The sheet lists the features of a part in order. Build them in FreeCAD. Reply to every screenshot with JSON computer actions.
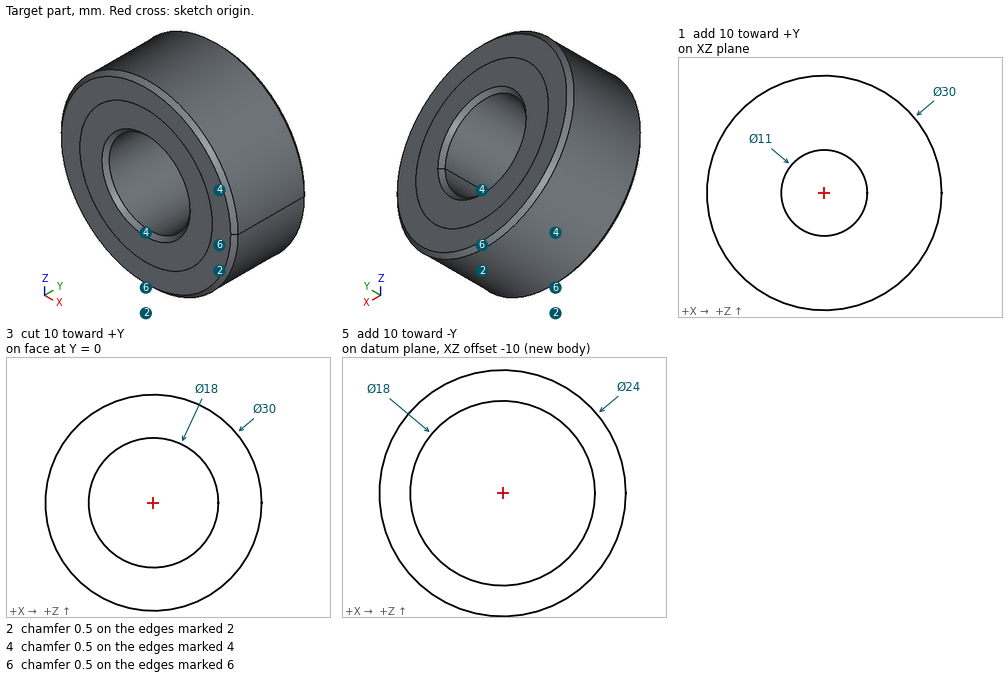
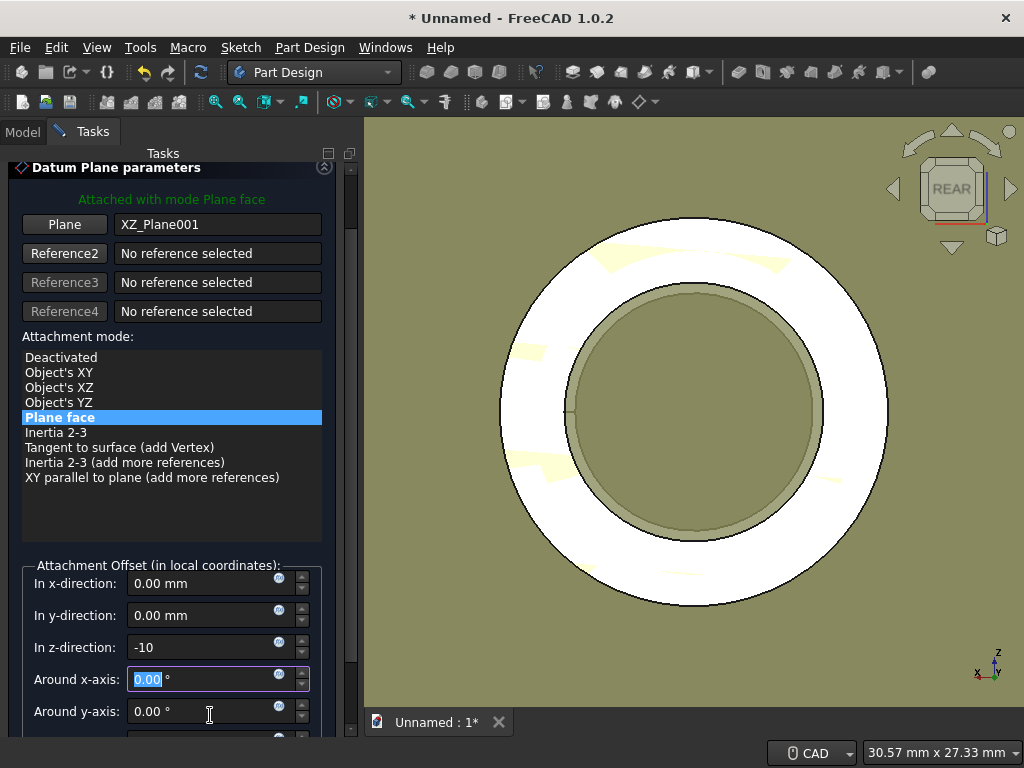
{"action": "scroll", "coordinate": [351, 450], "scroll_direction": "up", "scroll_amount": 2}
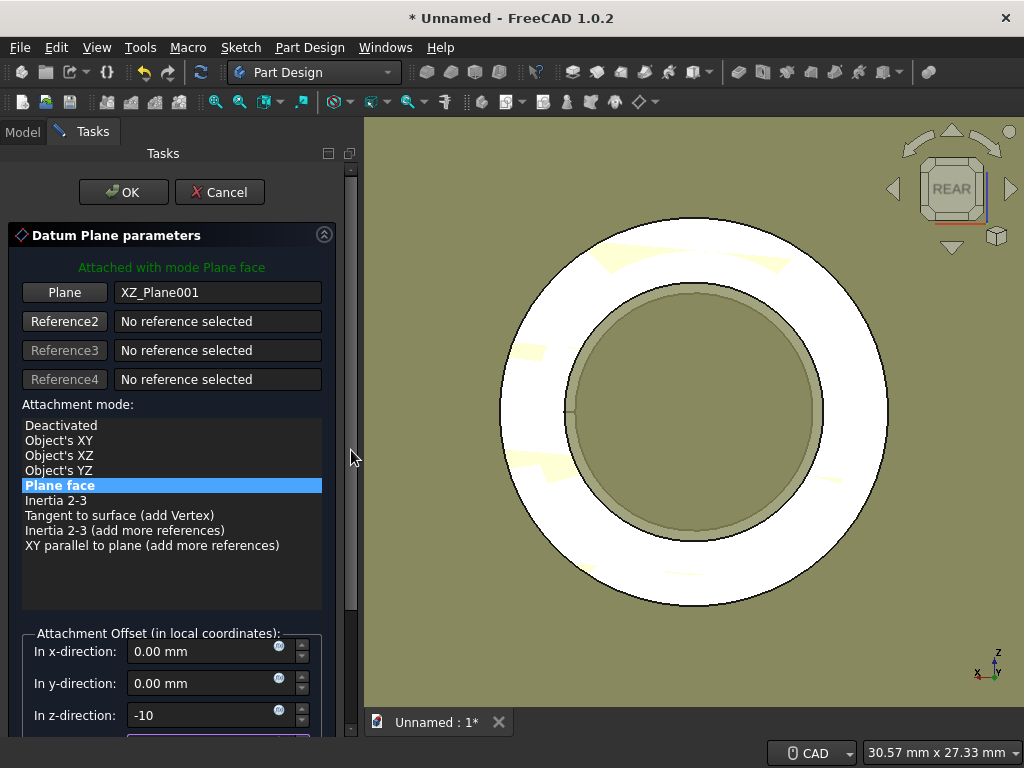
{"action": "left_click", "coordinate": [124, 192]}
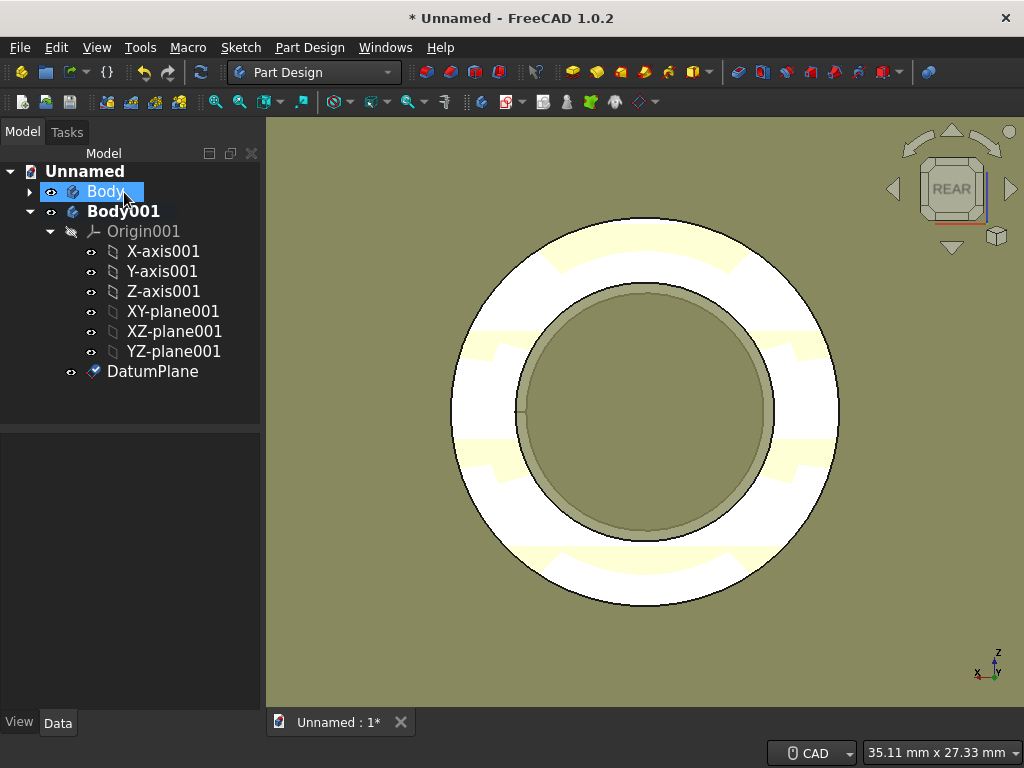
{"action": "left_click", "coordinate": [116, 372]}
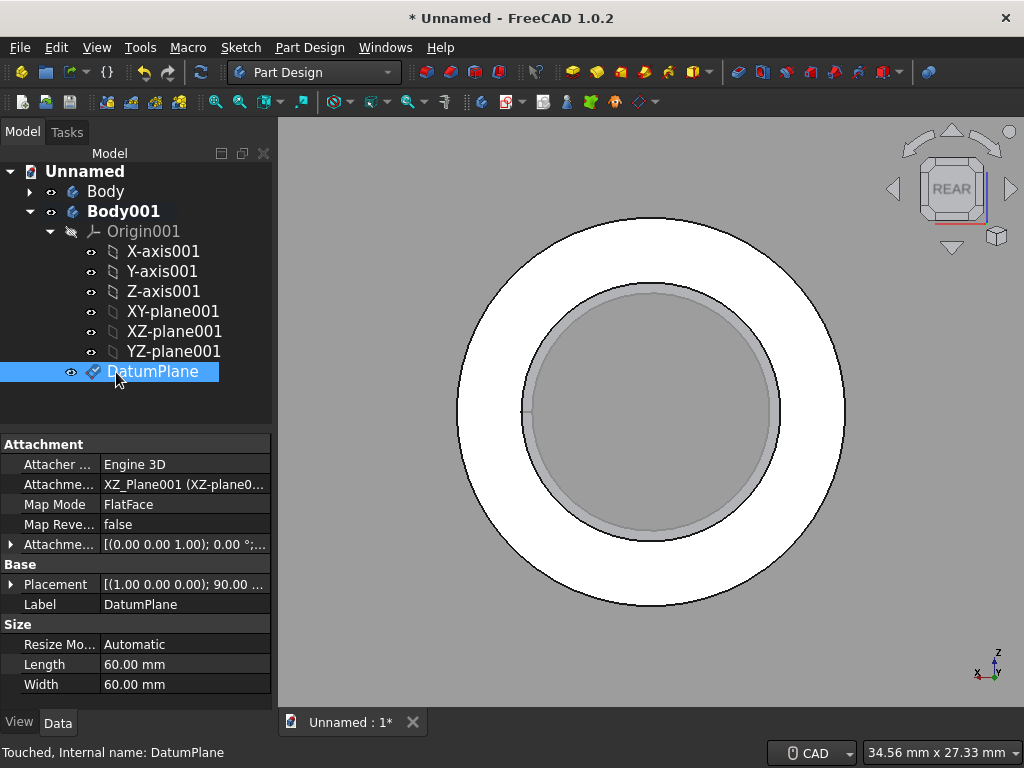
{"action": "left_click", "coordinate": [506, 102]}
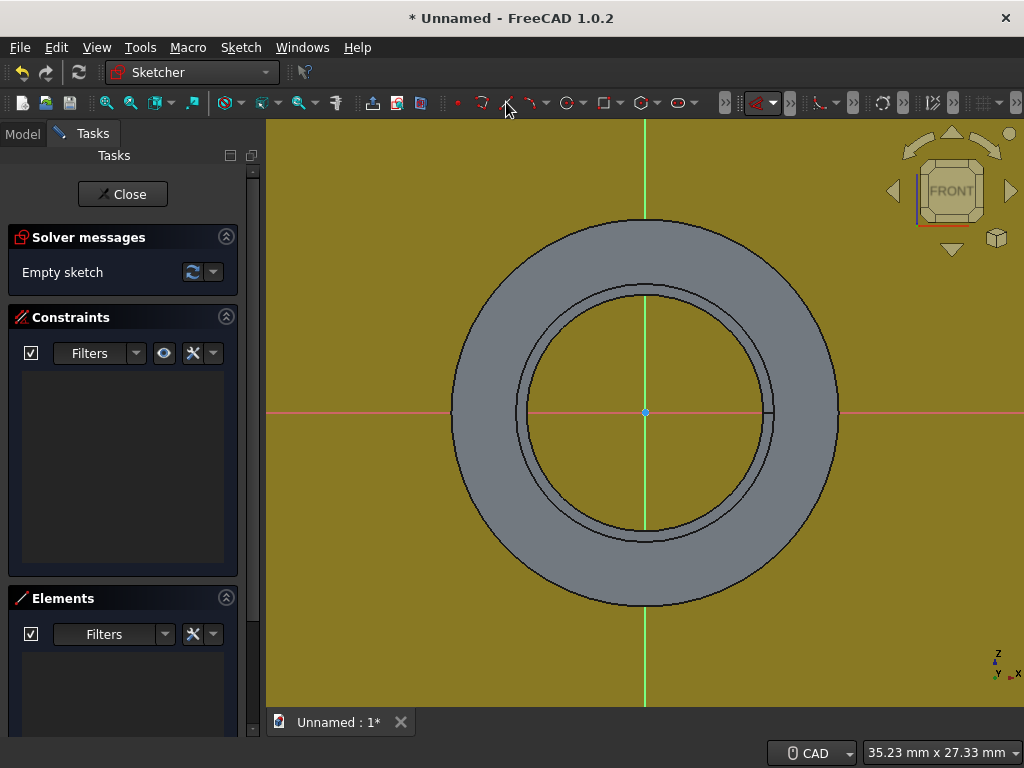
{"action": "scroll", "coordinate": [437, 413], "scroll_direction": "down", "scroll_amount": 2}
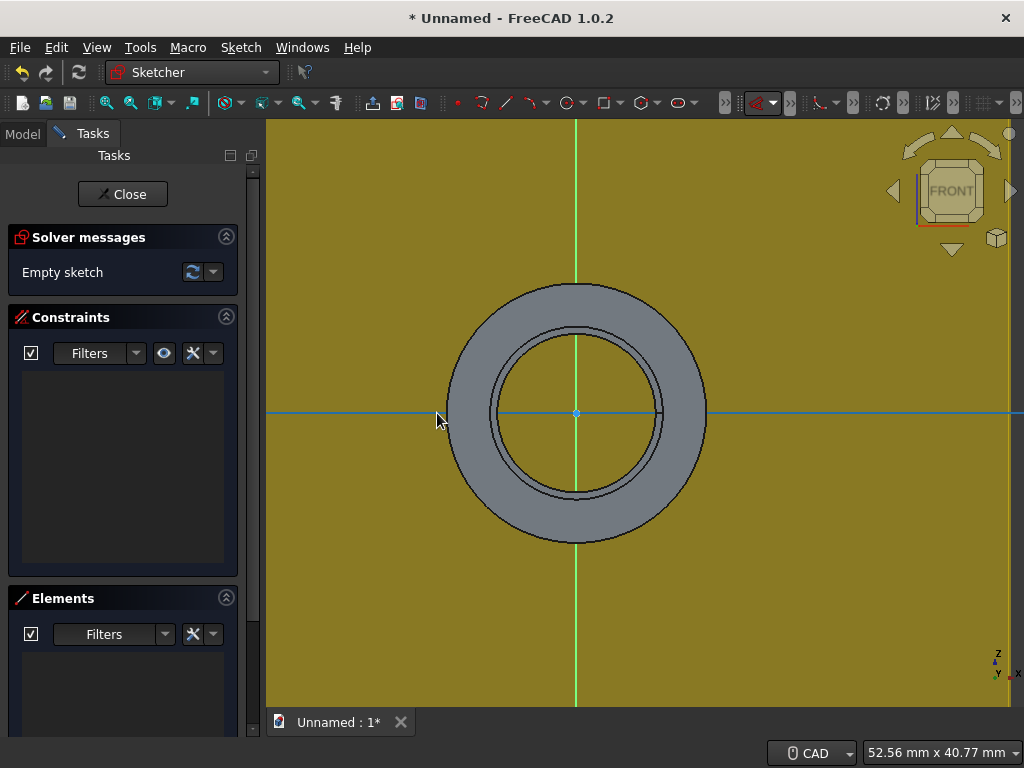
{"action": "left_click", "coordinate": [568, 104]}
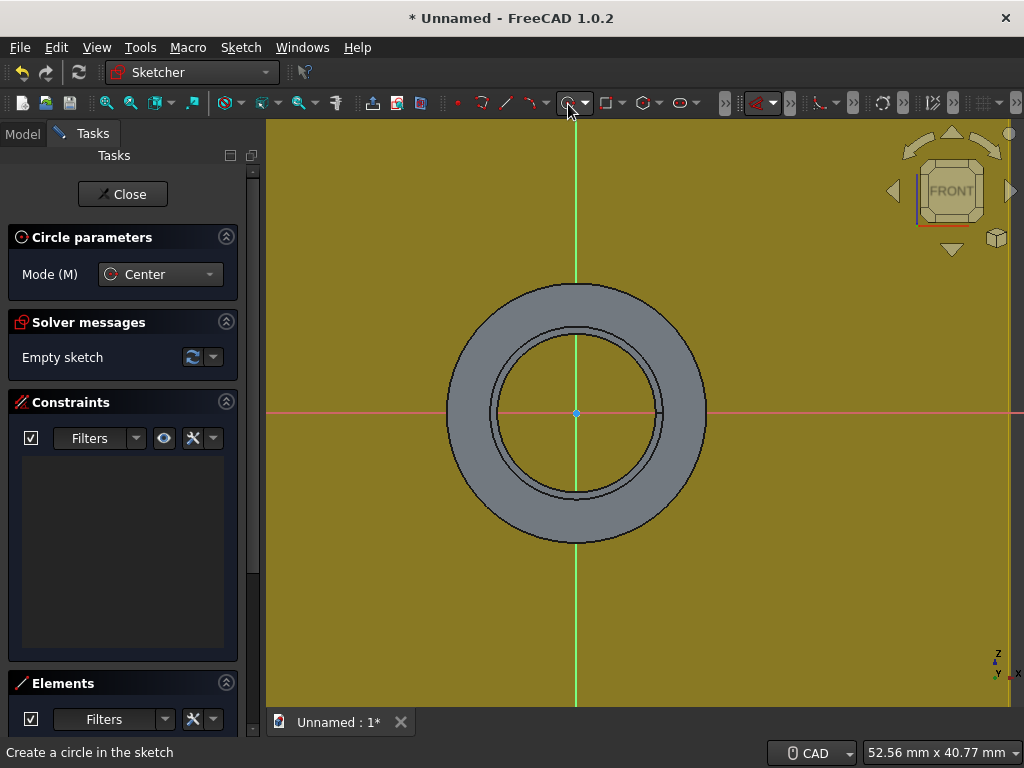
{"action": "left_click", "coordinate": [577, 413]}
{"action": "left_click", "coordinate": [699, 291]}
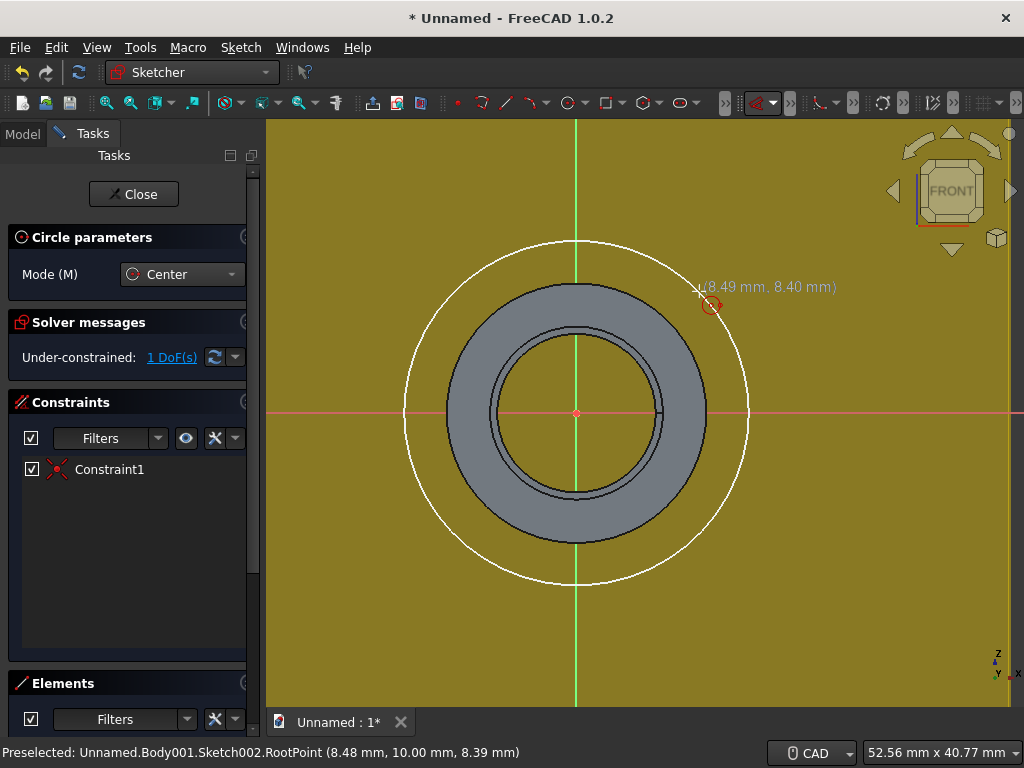
{"action": "left_click", "coordinate": [577, 413]}
{"action": "left_click", "coordinate": [668, 321]}
{"action": "key", "text": "Escape"}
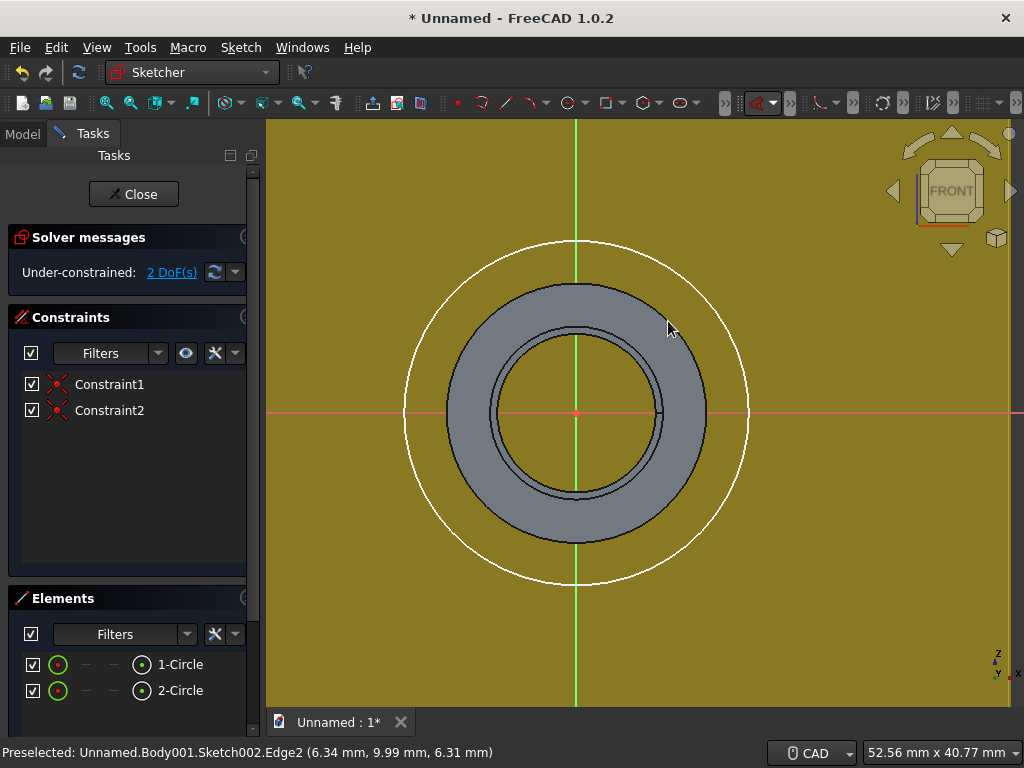
{"action": "left_click", "coordinate": [698, 291]}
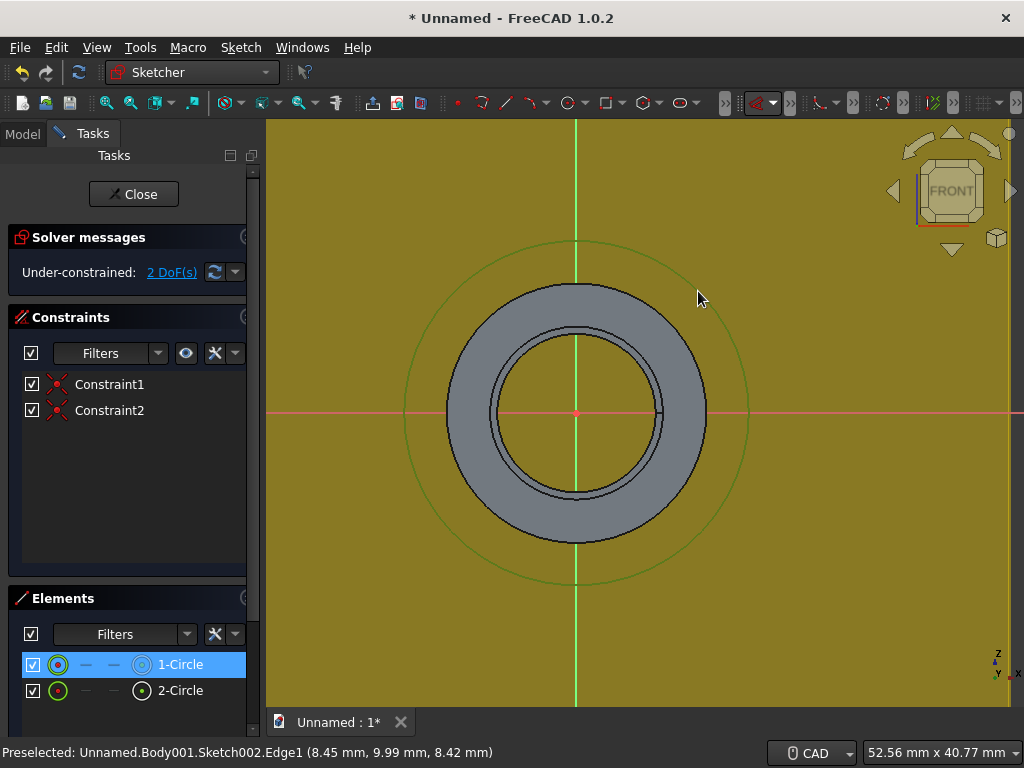
{"action": "left_click", "coordinate": [776, 104]}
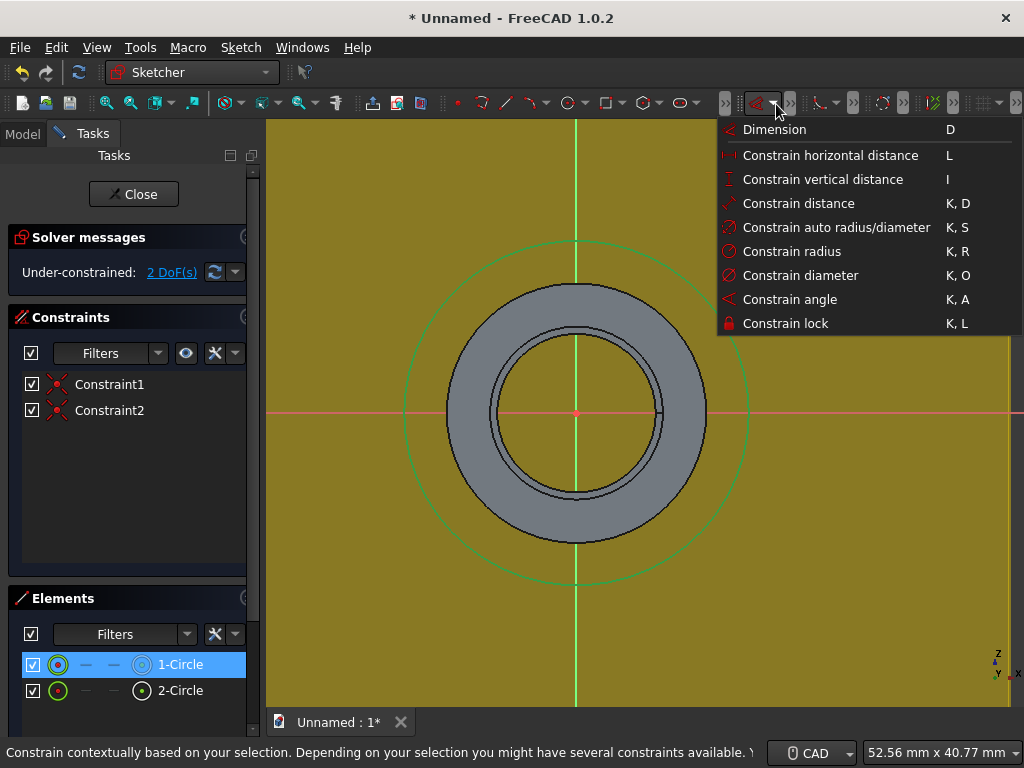
{"action": "left_click", "coordinate": [870, 275]}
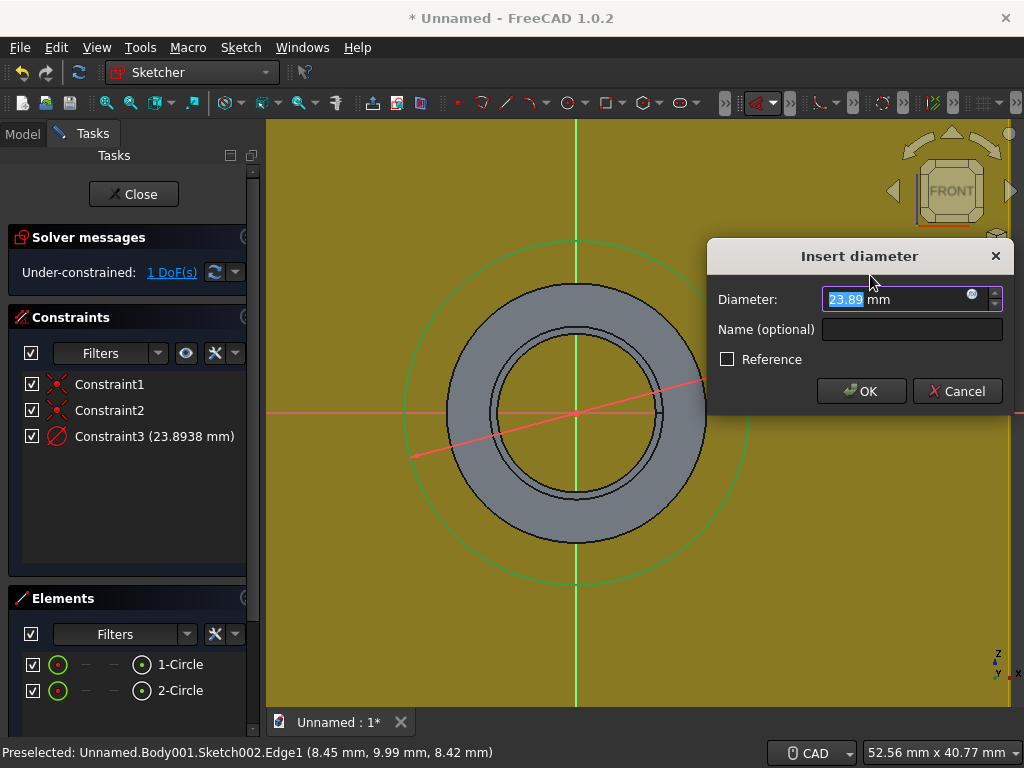
{"action": "type", "text": "24"}
{"action": "key", "text": "Return"}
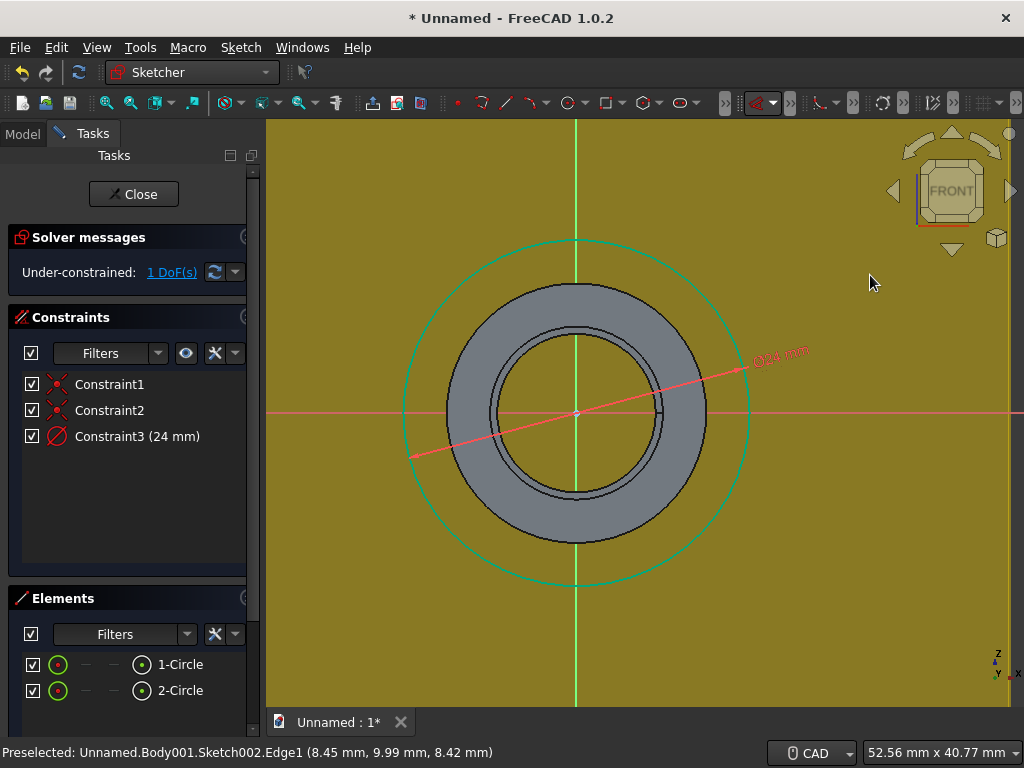
{"action": "left_click", "coordinate": [668, 322]}